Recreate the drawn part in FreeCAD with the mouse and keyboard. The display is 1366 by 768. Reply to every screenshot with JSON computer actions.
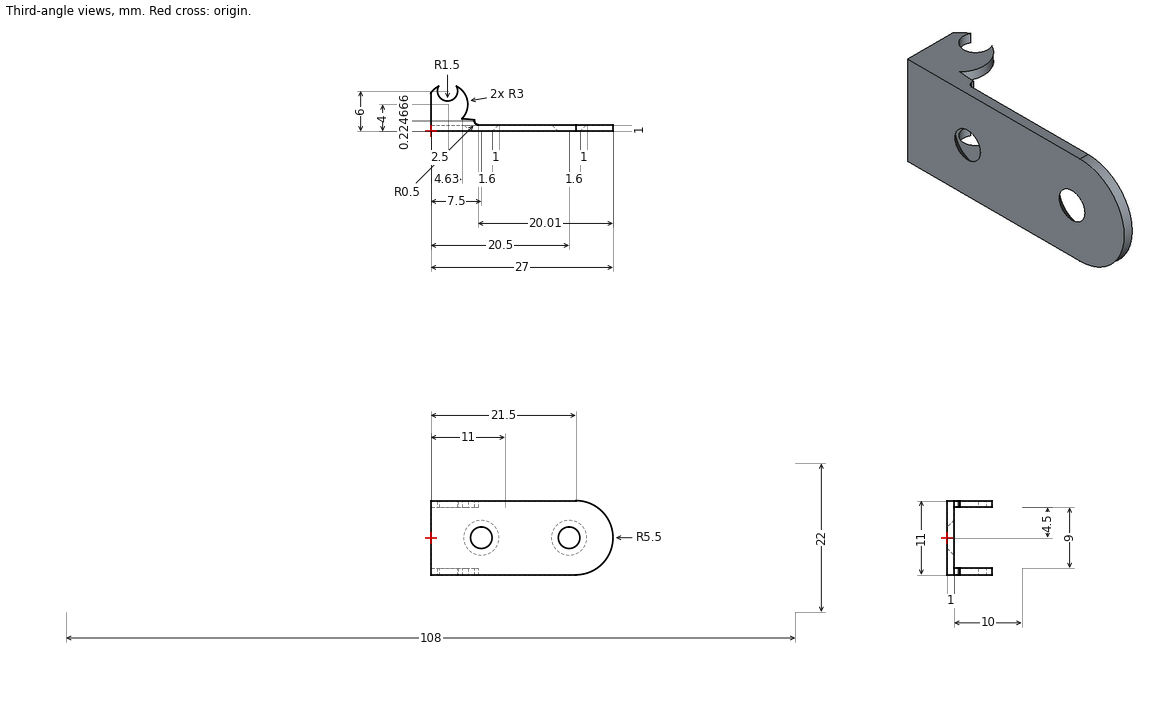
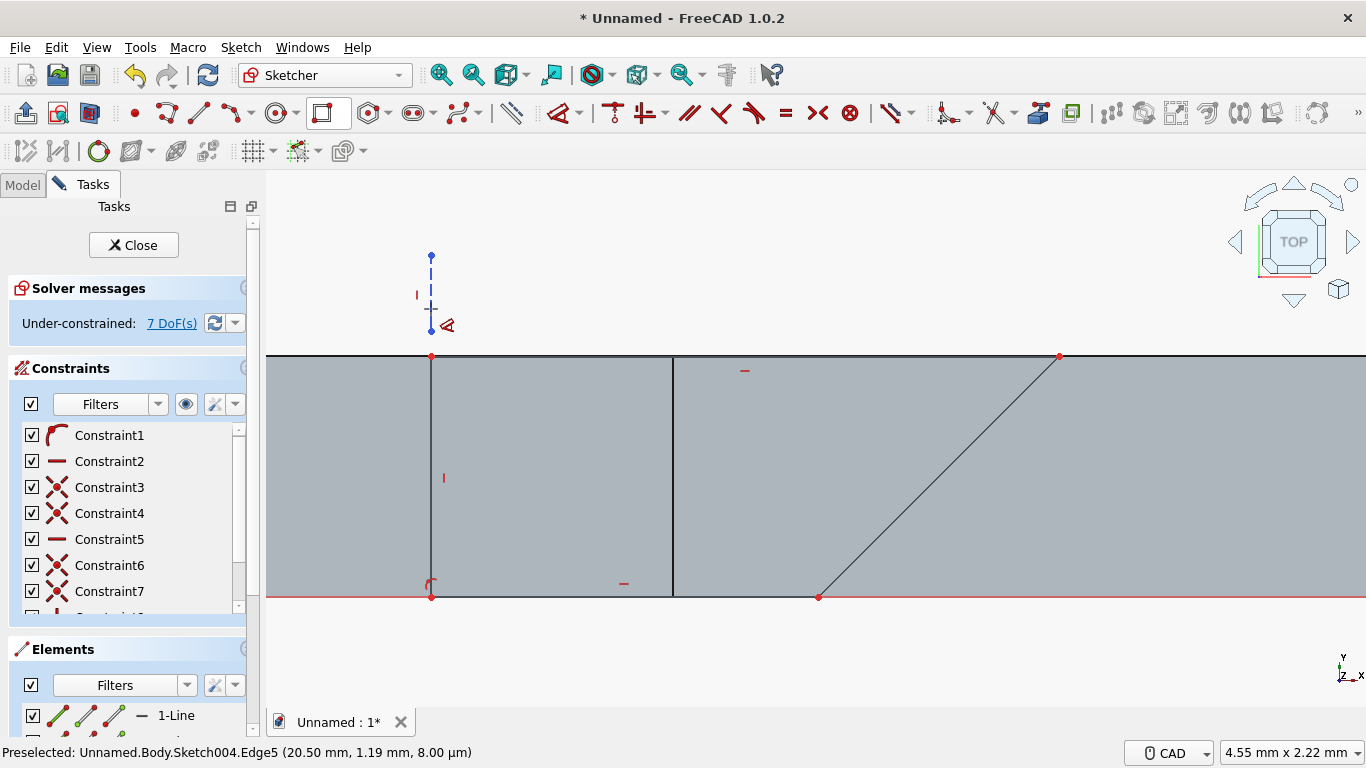
{"action": "left_click", "coordinate": [431, 429]}
{"action": "left_click", "coordinate": [397, 477]}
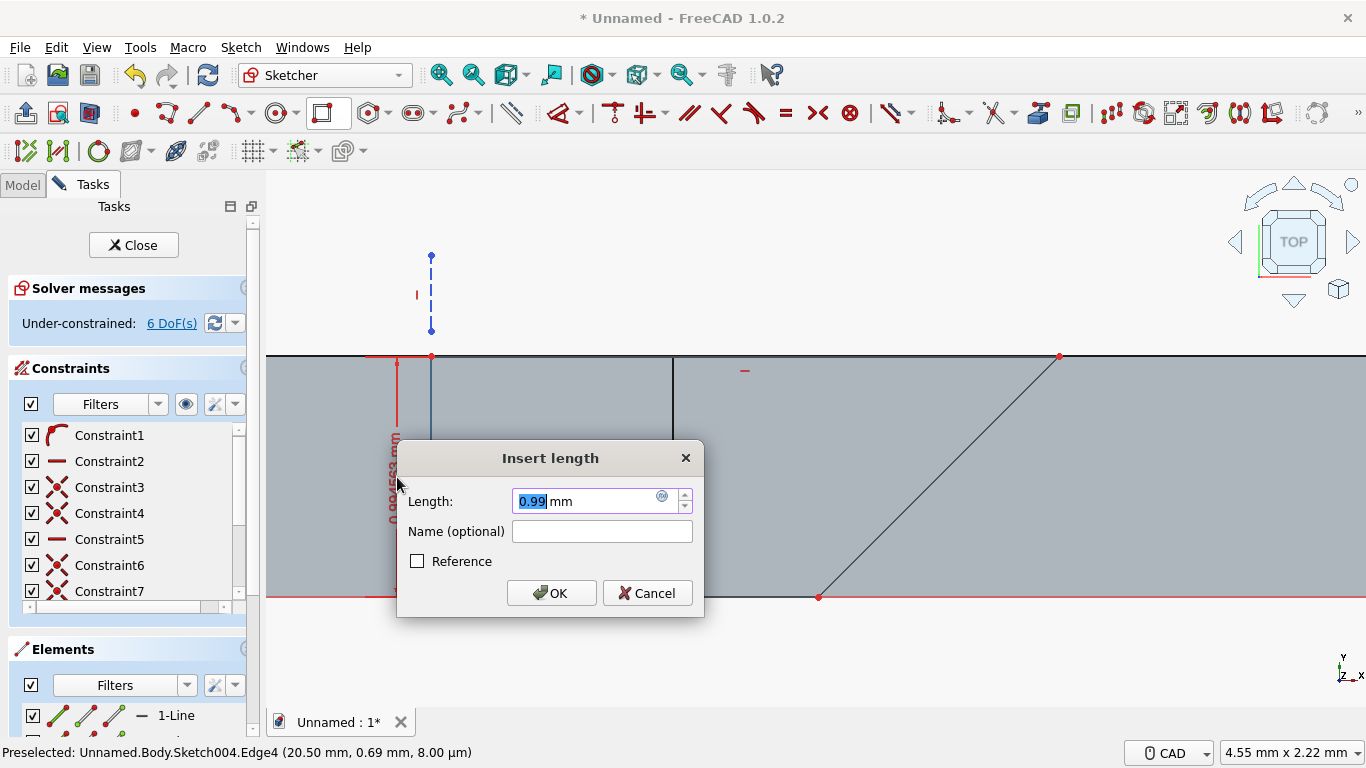
{"action": "type", "text": "1"}
{"action": "key", "text": "Return"}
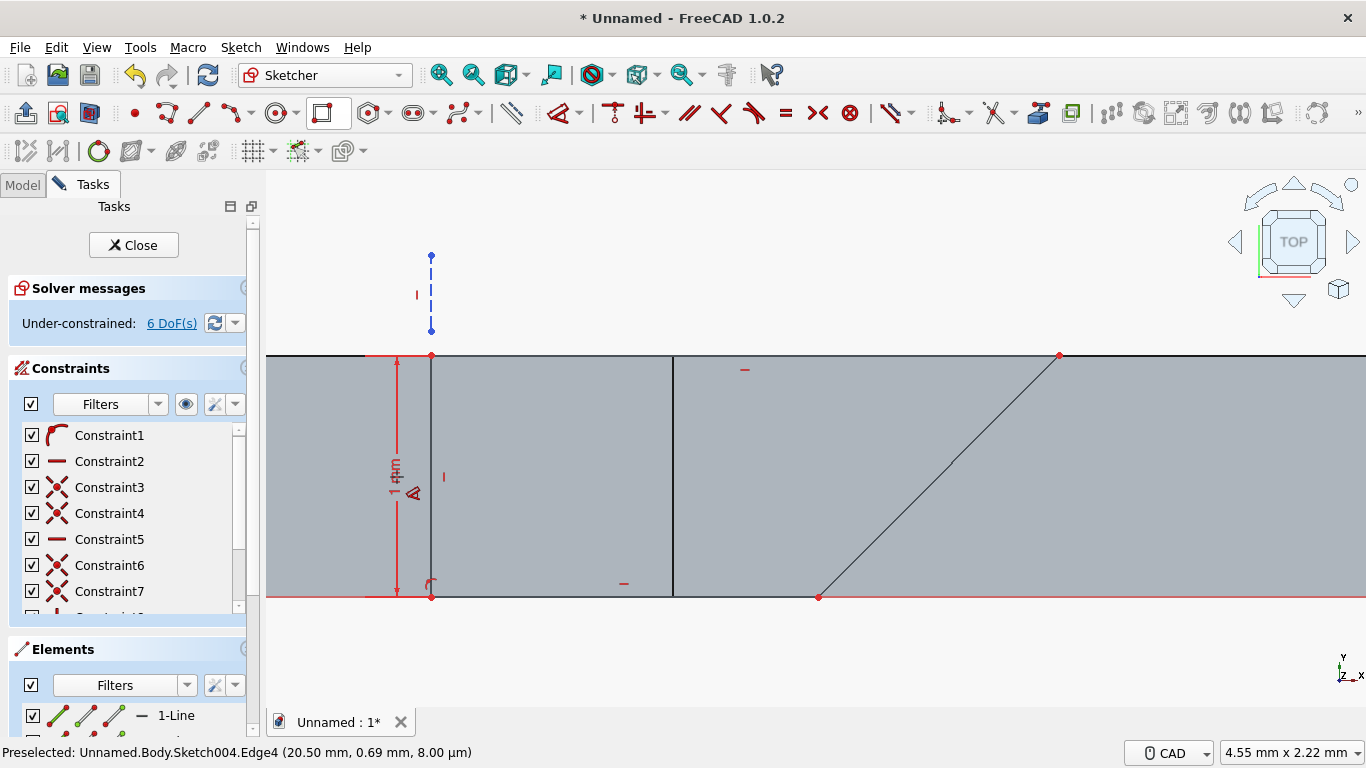
{"action": "left_click", "coordinate": [890, 525]}
{"action": "left_click", "coordinate": [938, 631]}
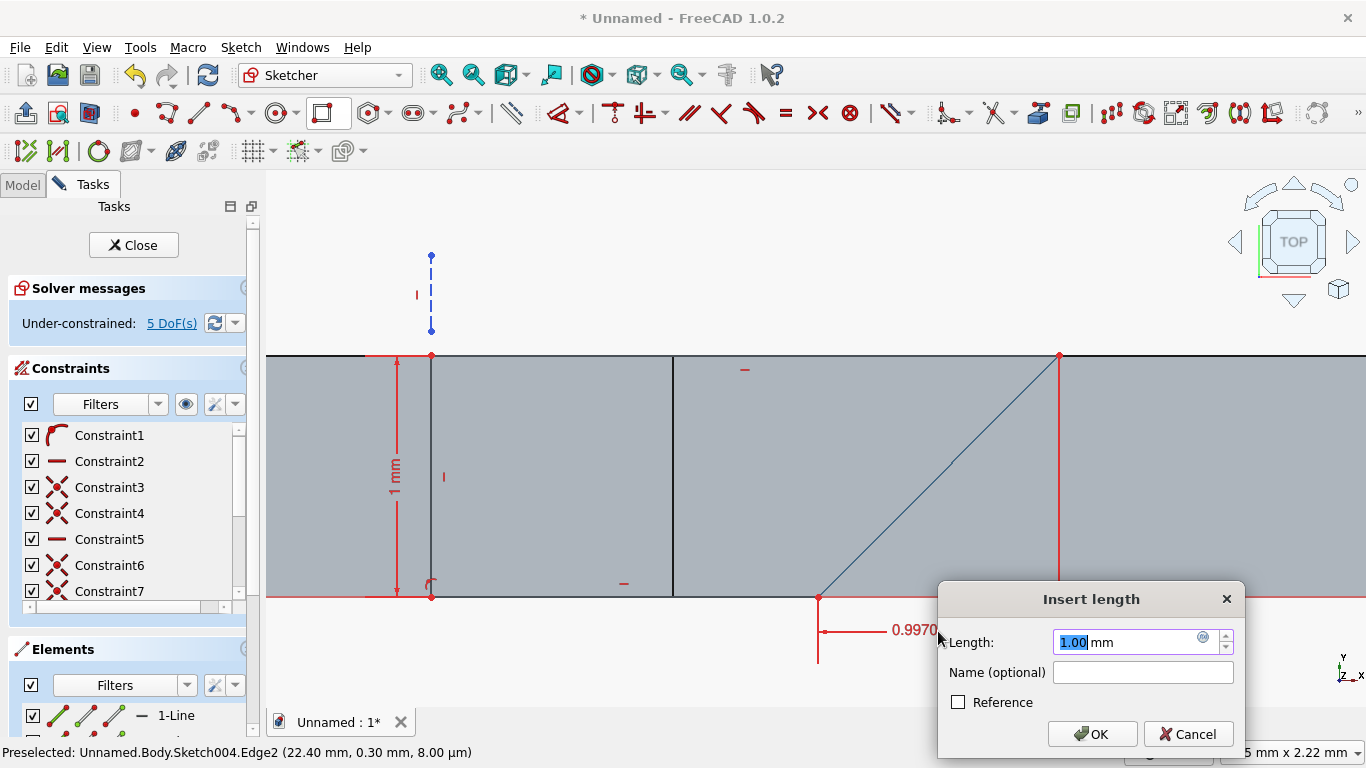
{"action": "type", "text": "1"}
{"action": "key", "text": "Return"}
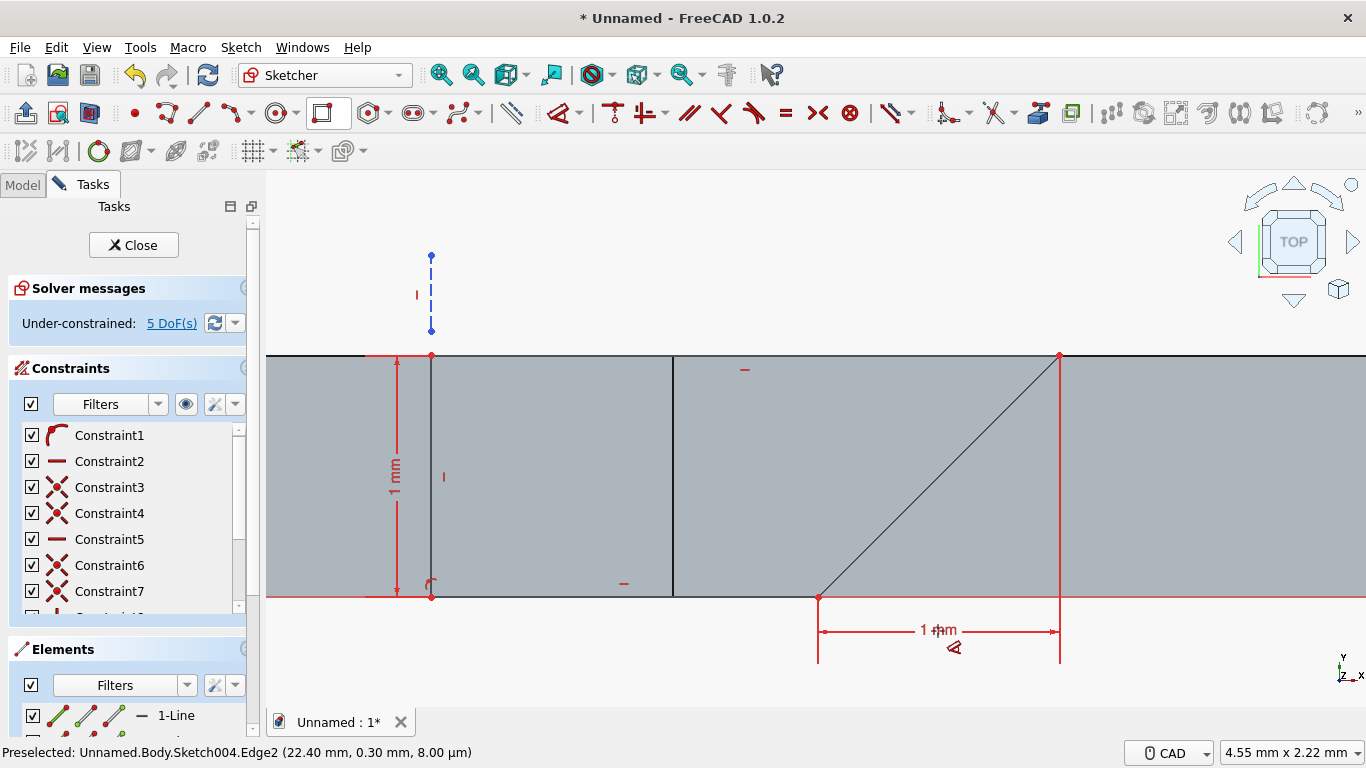
{"action": "left_click", "coordinate": [547, 597]}
{"action": "left_click", "coordinate": [625, 631]}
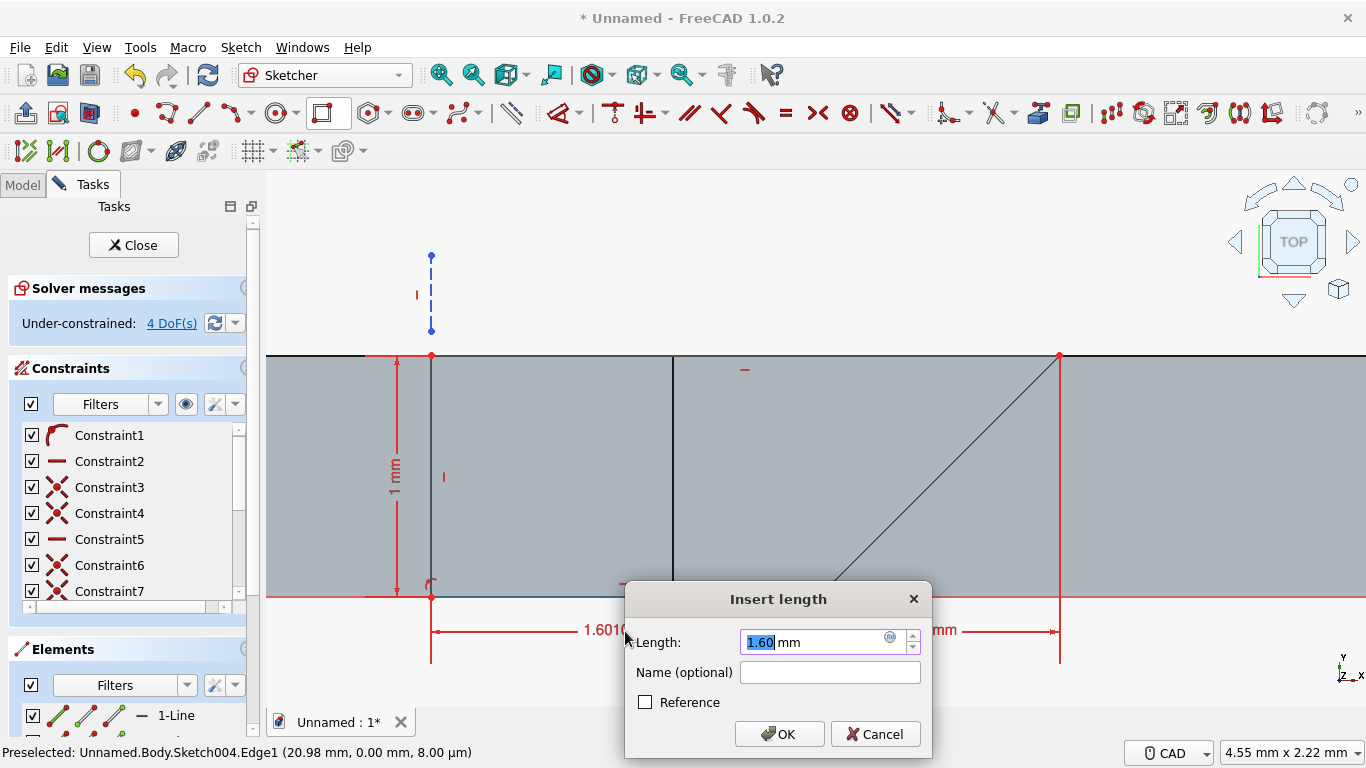
{"action": "type", "text": "1.6"}
{"action": "key", "text": "Return"}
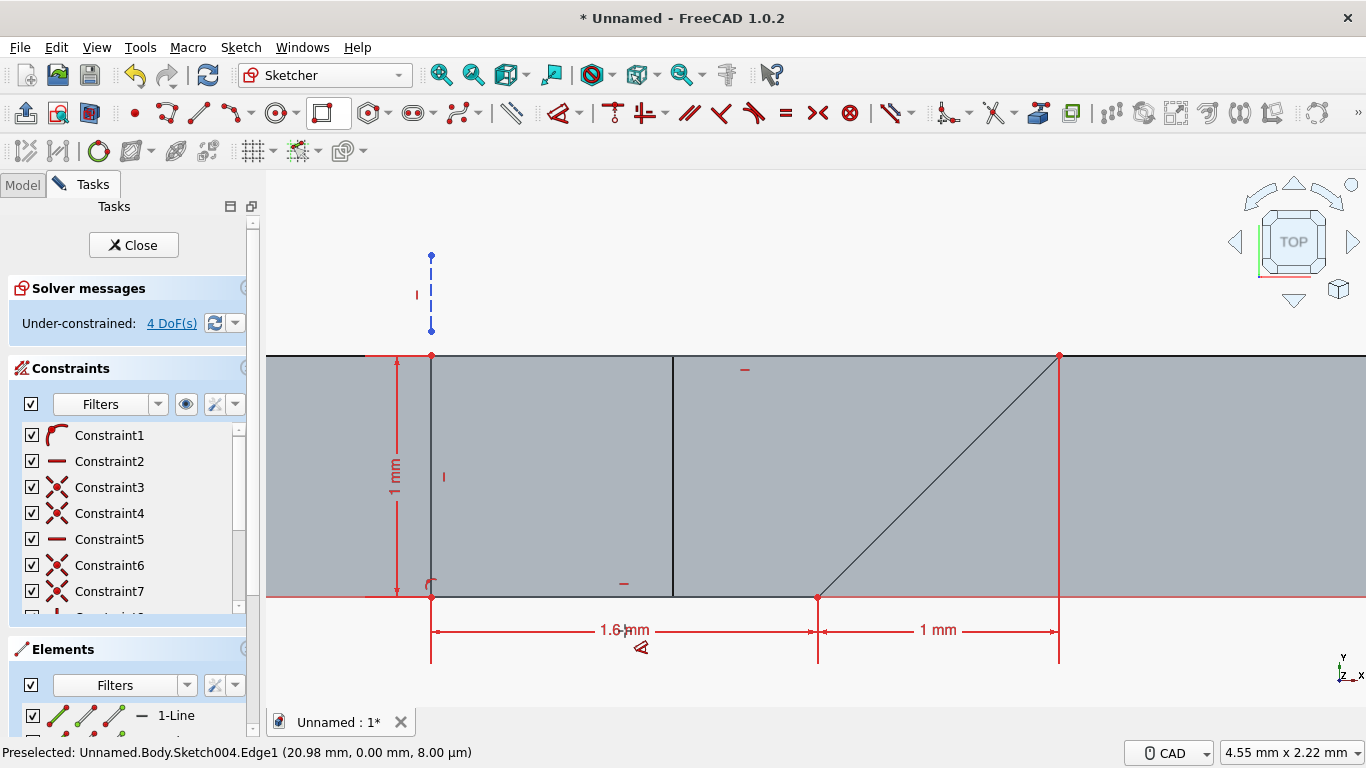
{"action": "left_click", "coordinate": [431, 597]}
{"action": "left_click", "coordinate": [363, 631]}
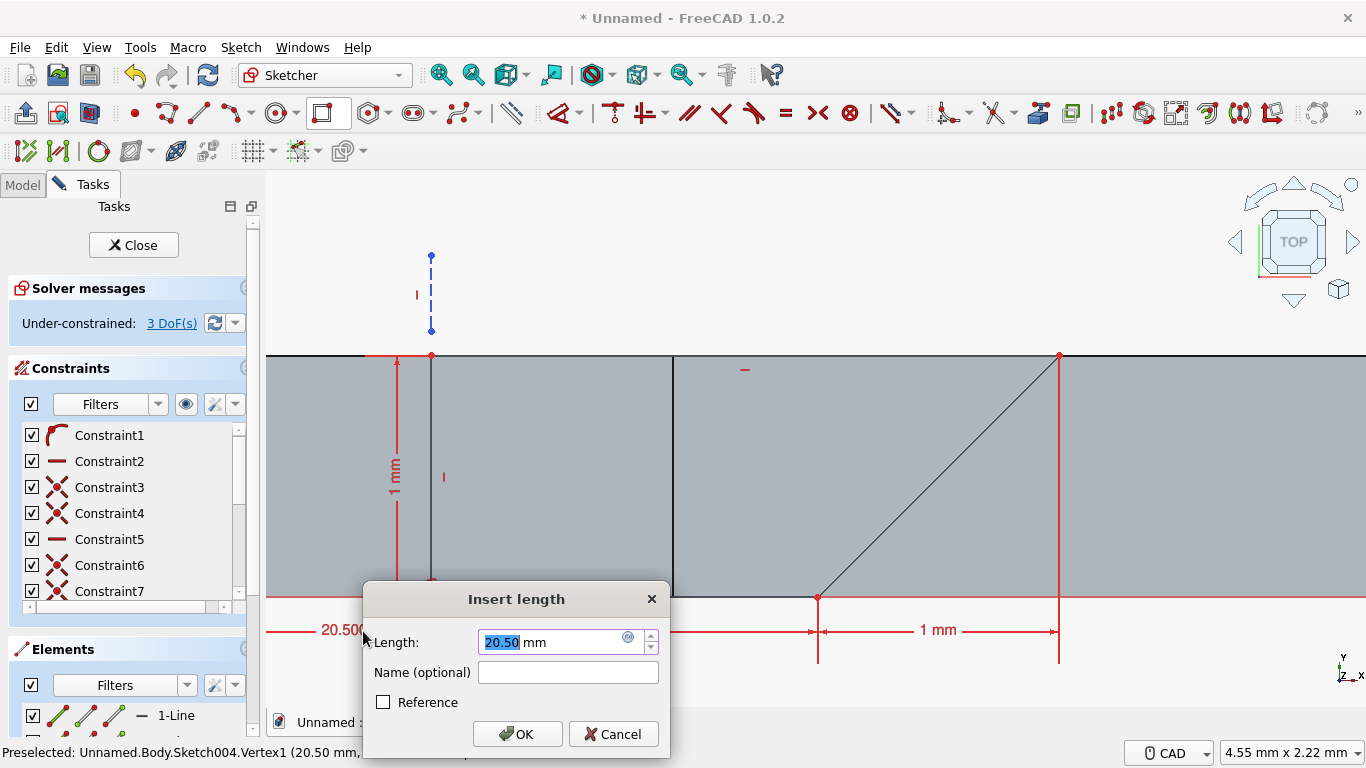
{"action": "type", "text": "20.5"}
{"action": "key", "text": "Return"}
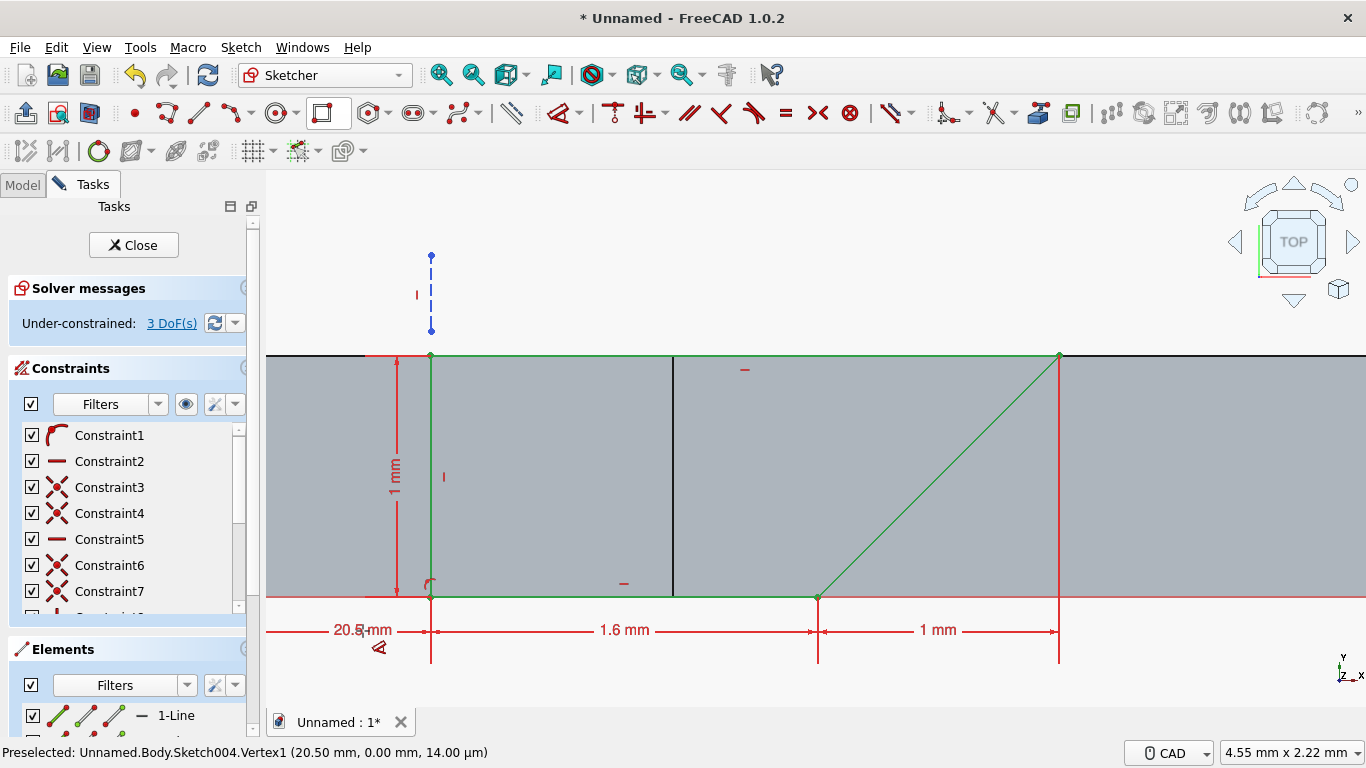
{"action": "left_click", "coordinate": [431, 332]}
{"action": "left_click", "coordinate": [363, 298]}